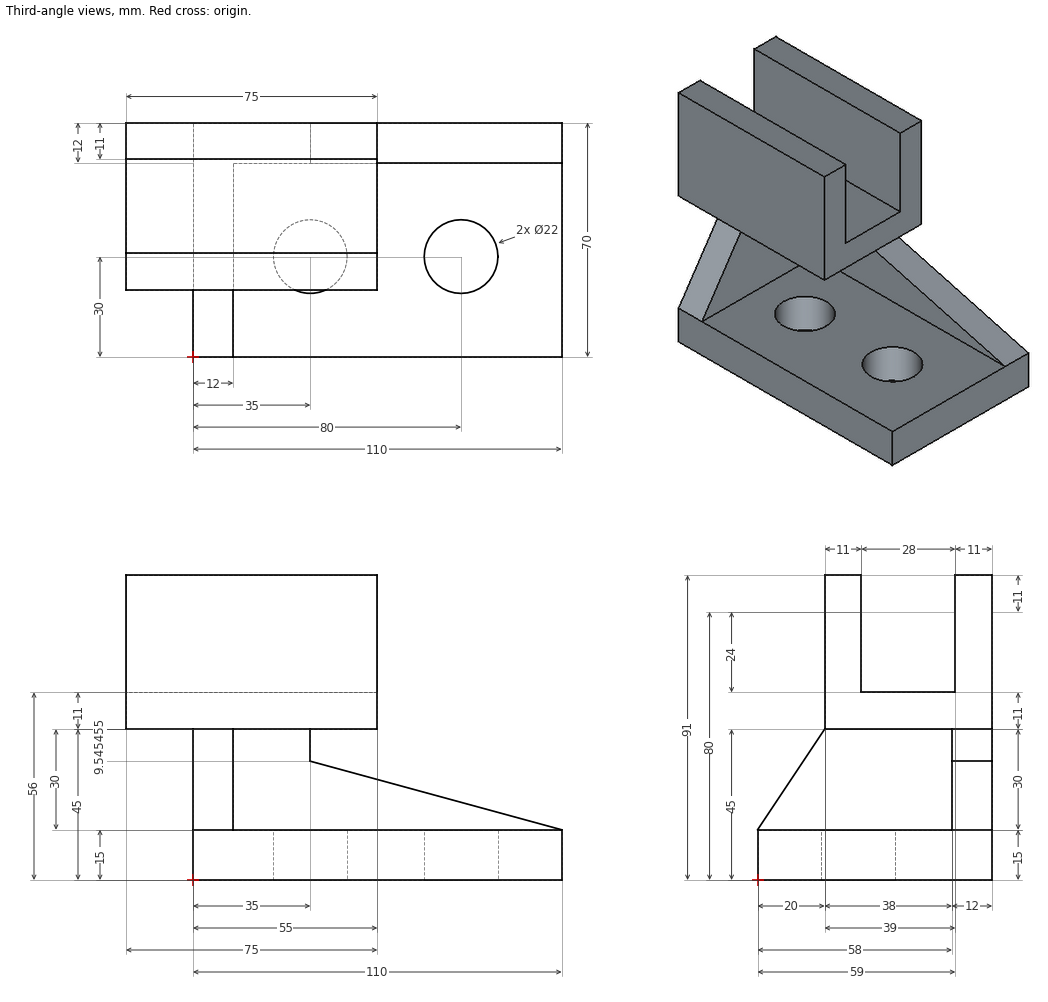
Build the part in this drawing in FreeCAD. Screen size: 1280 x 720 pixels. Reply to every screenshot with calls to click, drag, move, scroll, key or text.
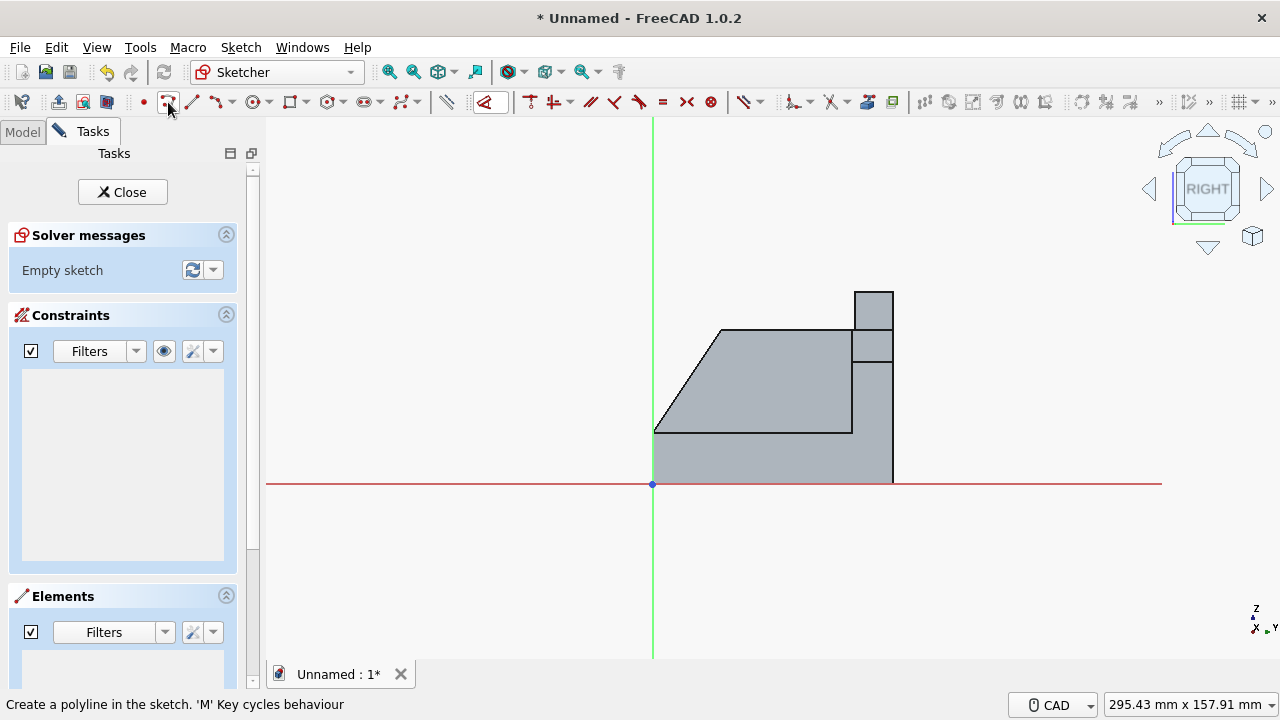
click(722, 330)
click(855, 330)
click(855, 292)
click(759, 292)
click(759, 210)
click(722, 210)
click(722, 331)
key(Escape)
key(Escape)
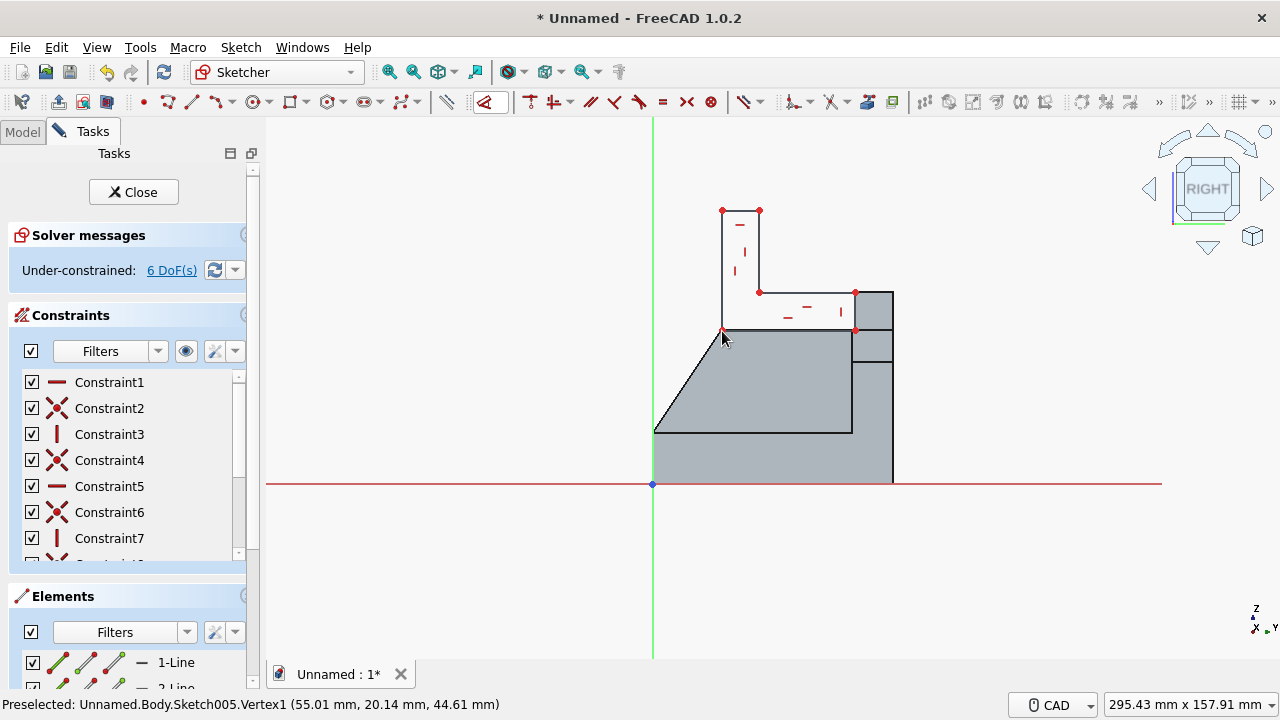
click(762, 331)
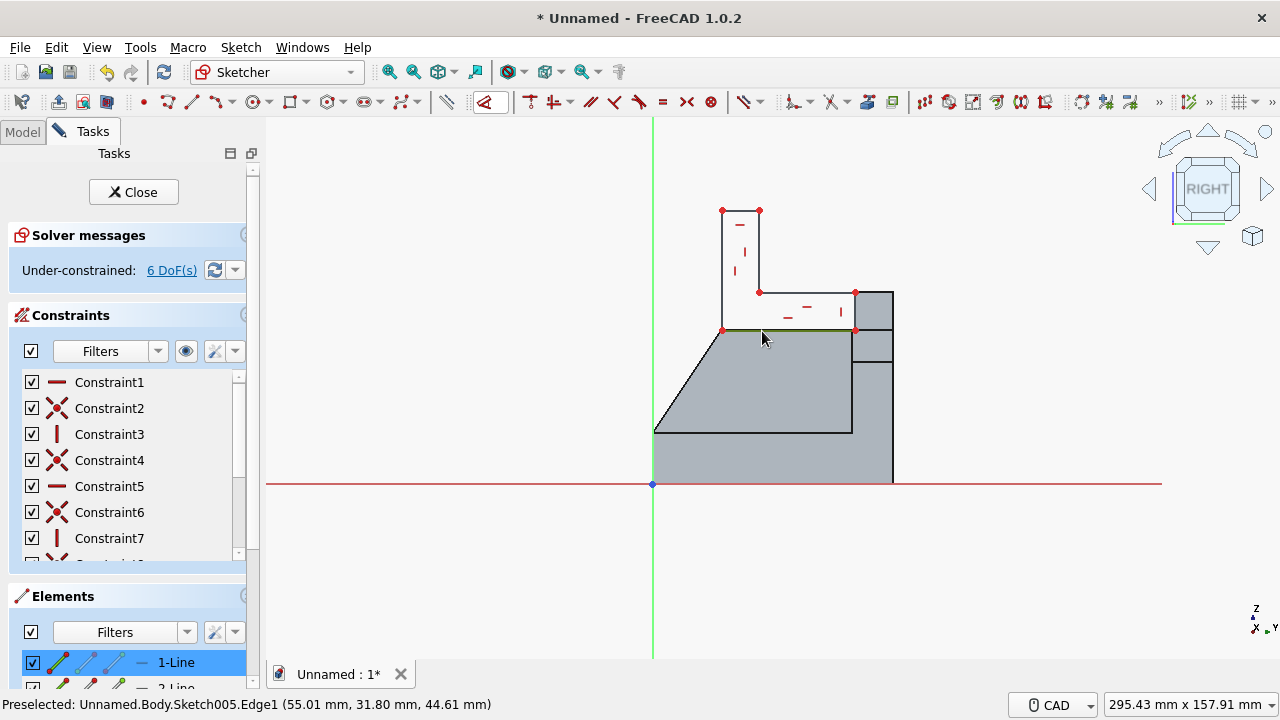
click(502, 102)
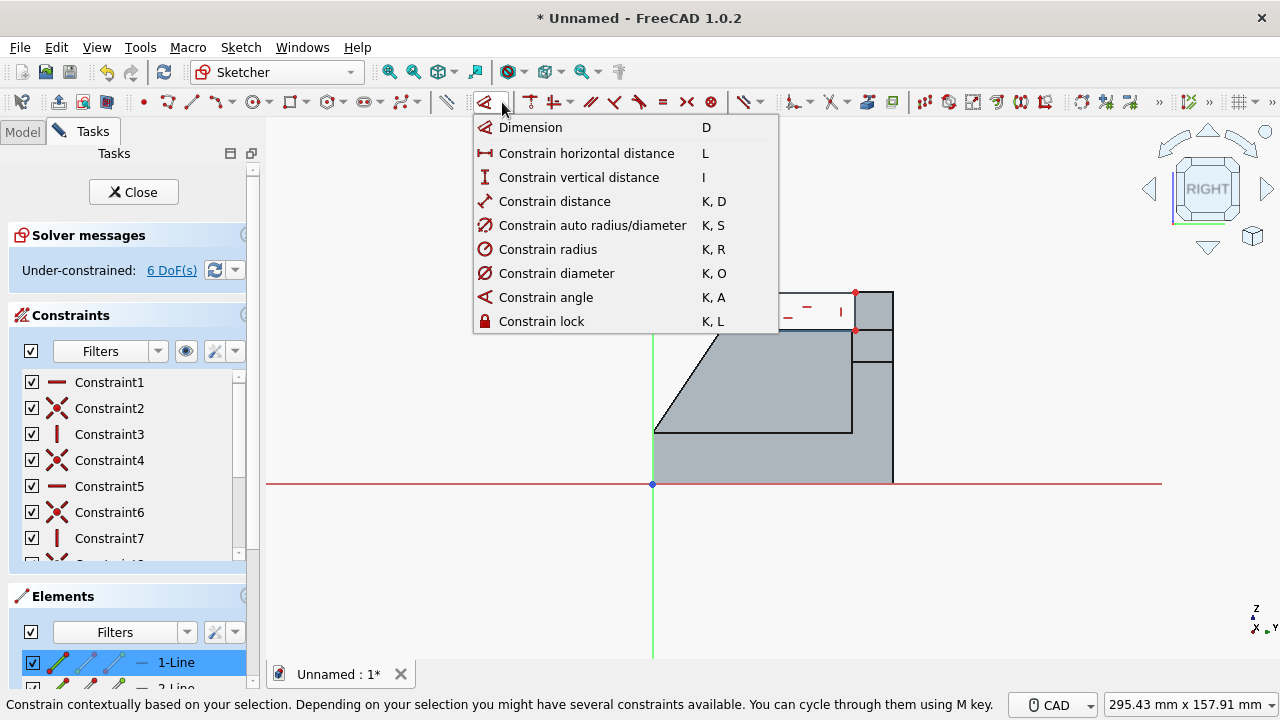
click(626, 153)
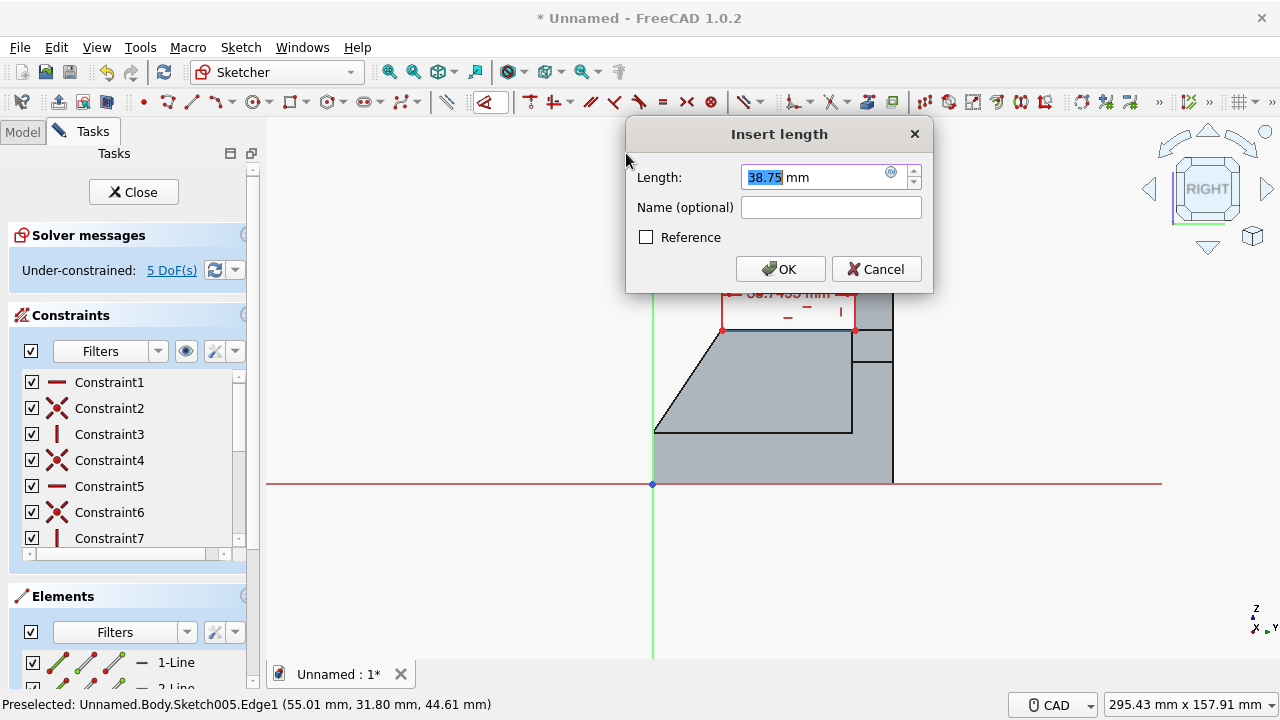
text(39)
key(Return)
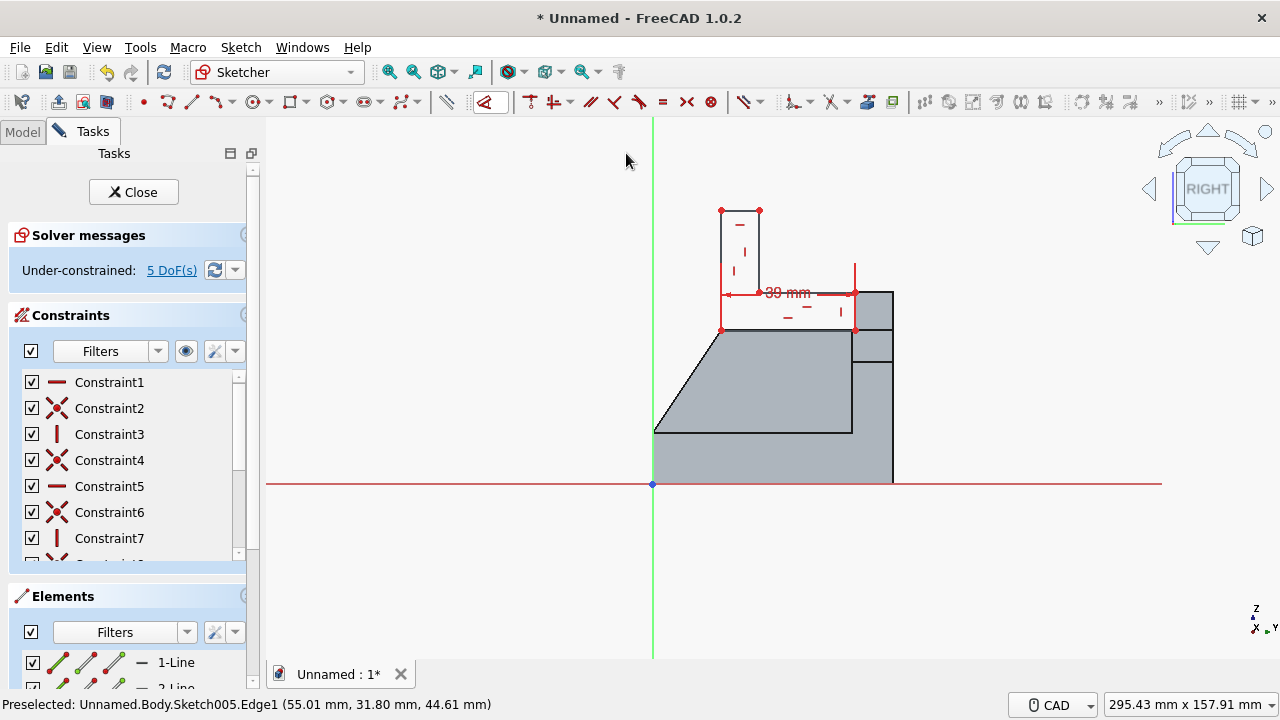
click(855, 320)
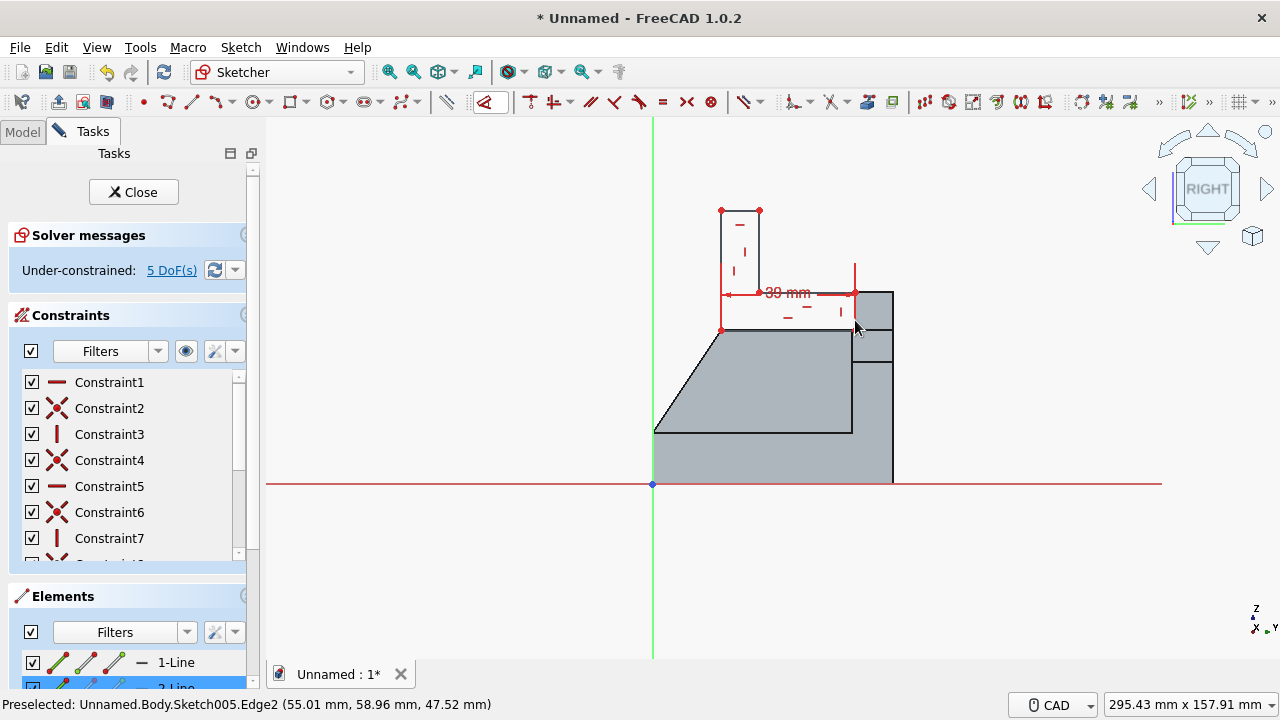
click(502, 102)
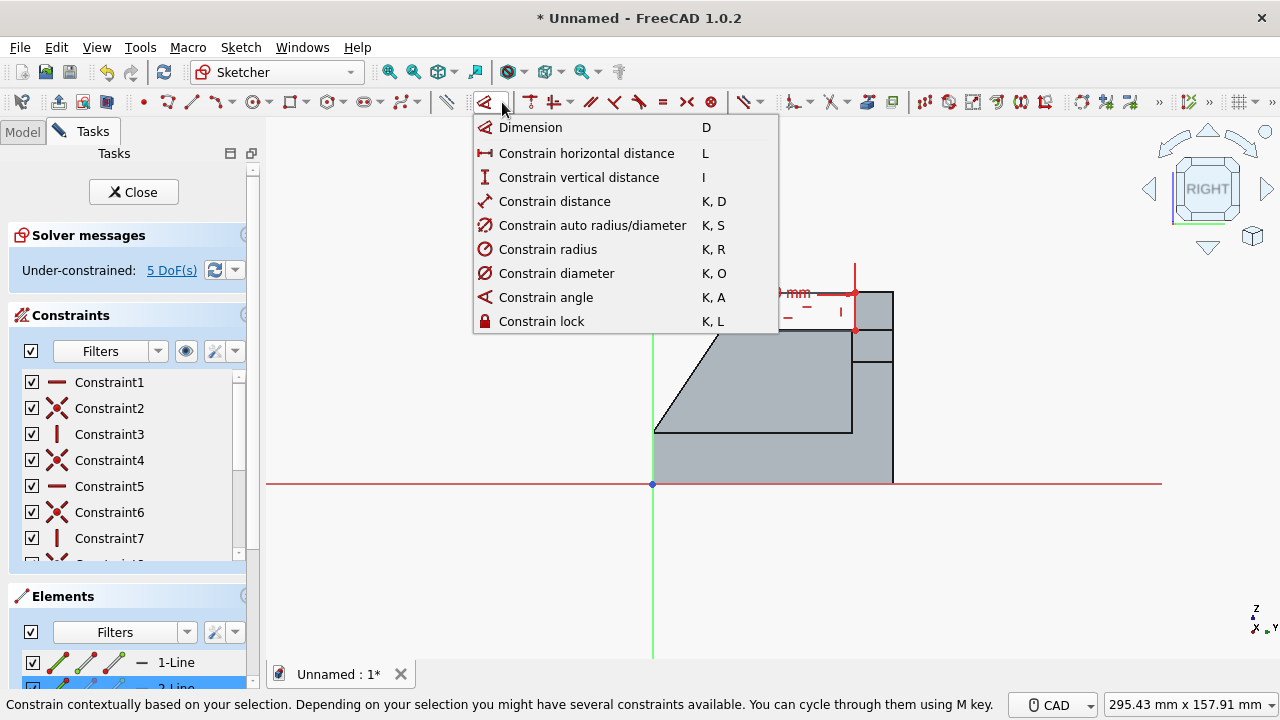
click(626, 177)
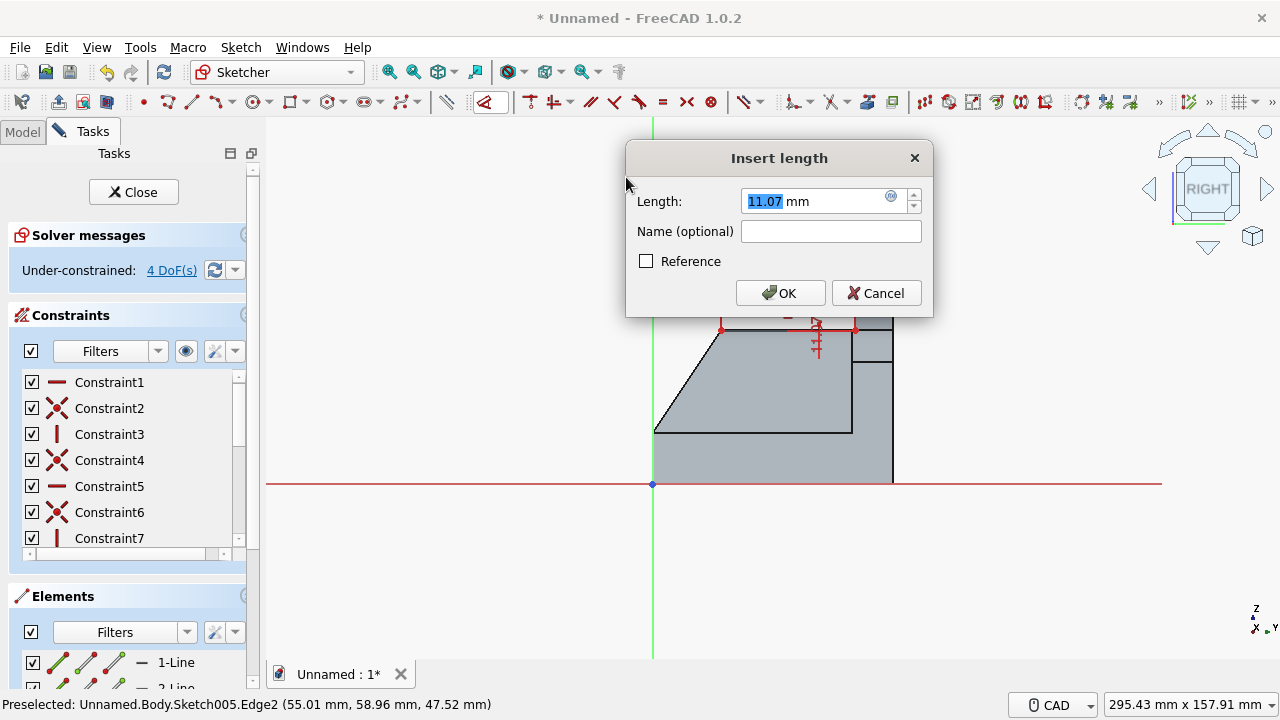
text(11)
key(Return)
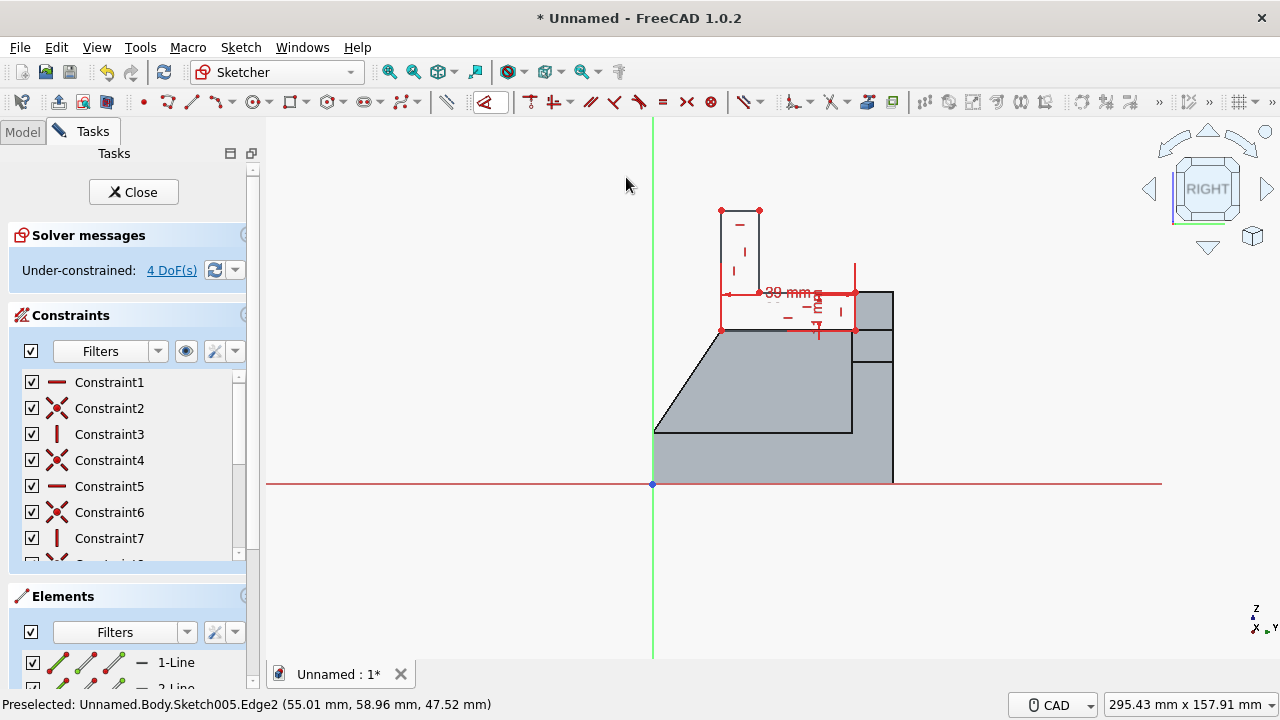
click(836, 293)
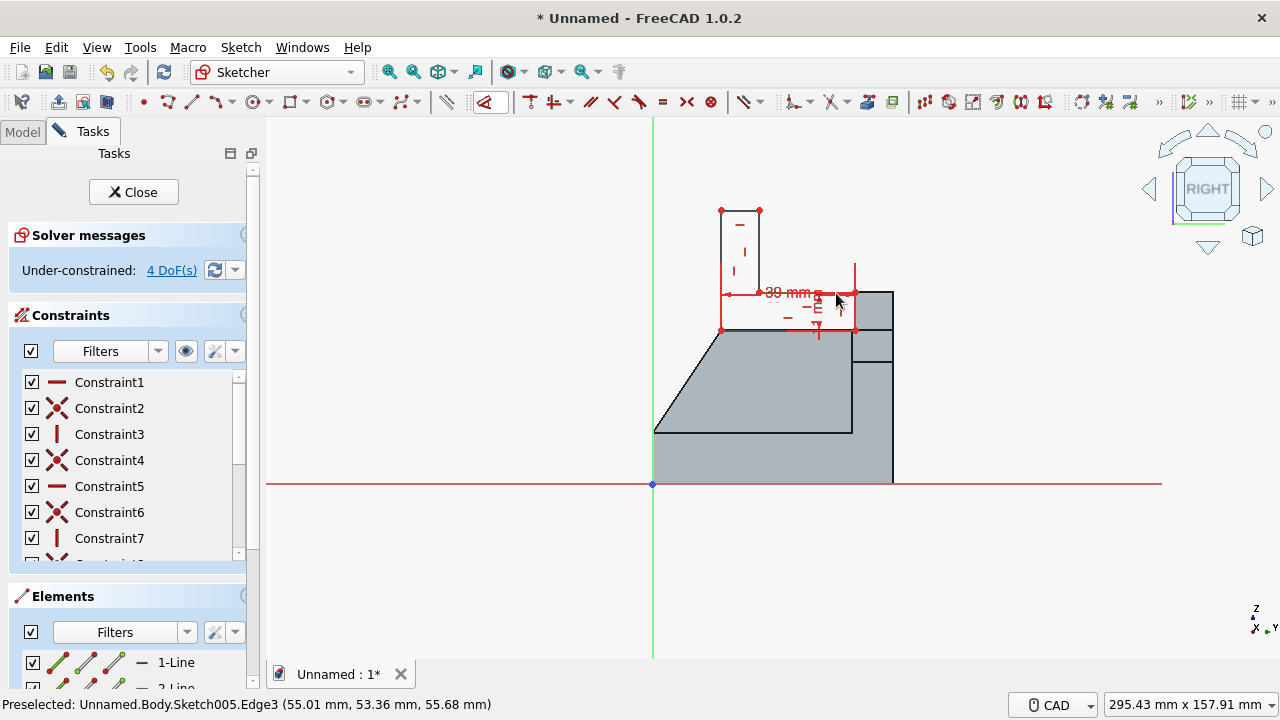
click(502, 102)